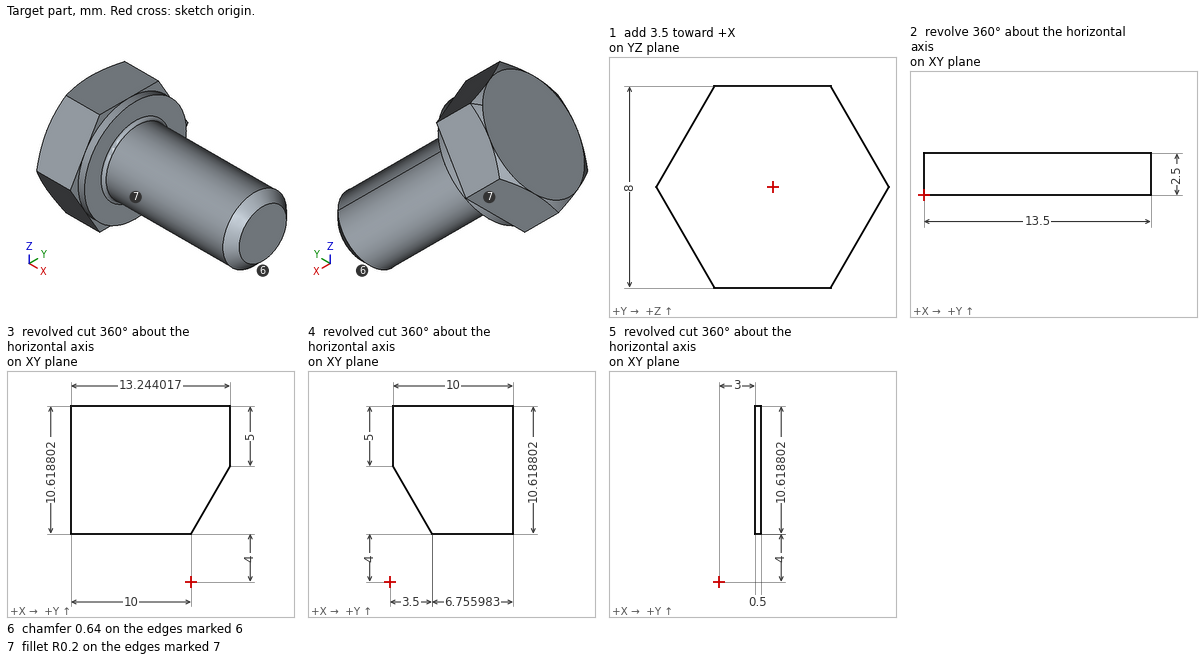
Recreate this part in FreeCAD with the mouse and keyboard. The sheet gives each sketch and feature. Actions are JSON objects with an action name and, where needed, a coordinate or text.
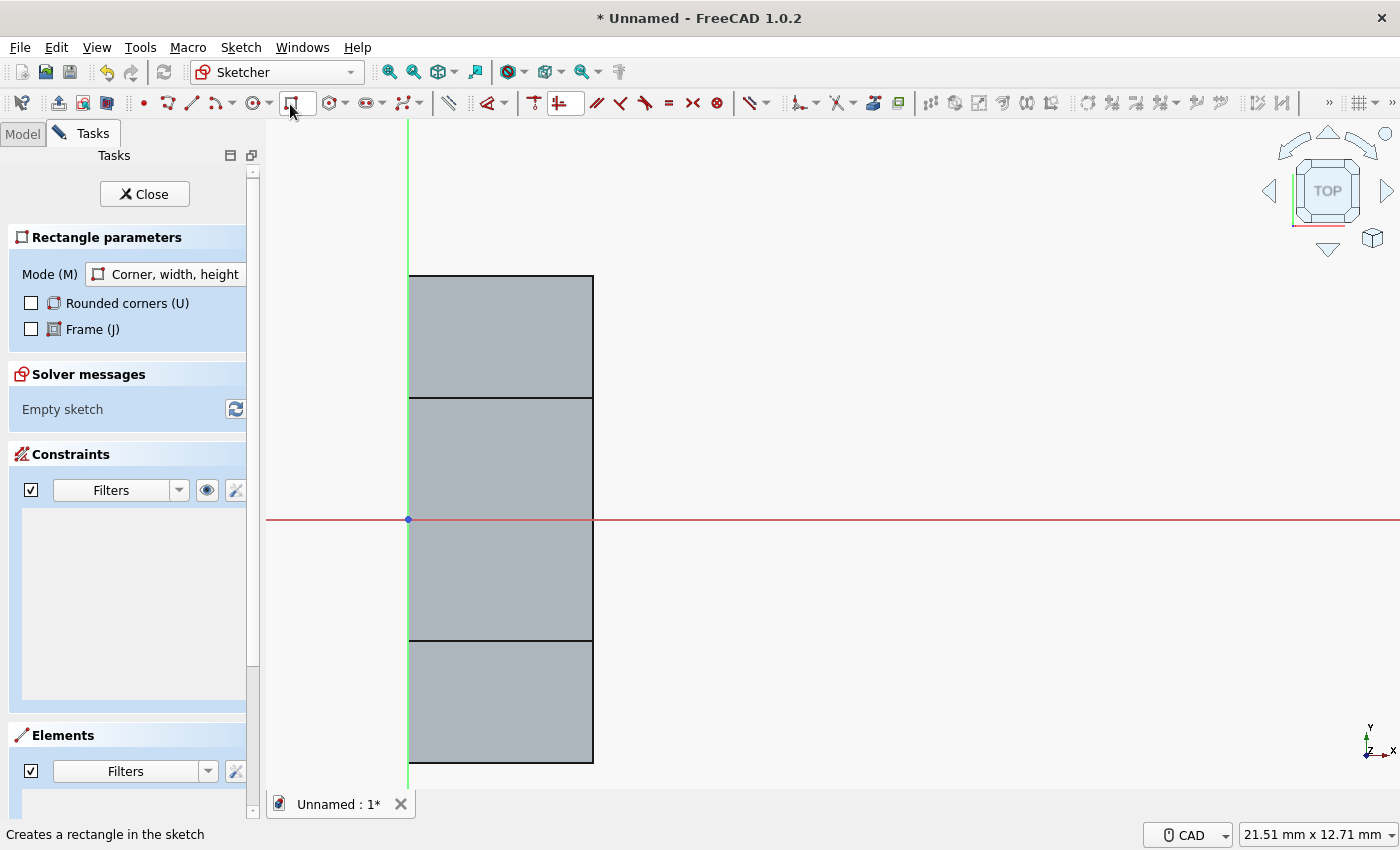
{"action": "left_click", "coordinate": [408, 520]}
{"action": "mouse_move", "coordinate": [1120, 388]}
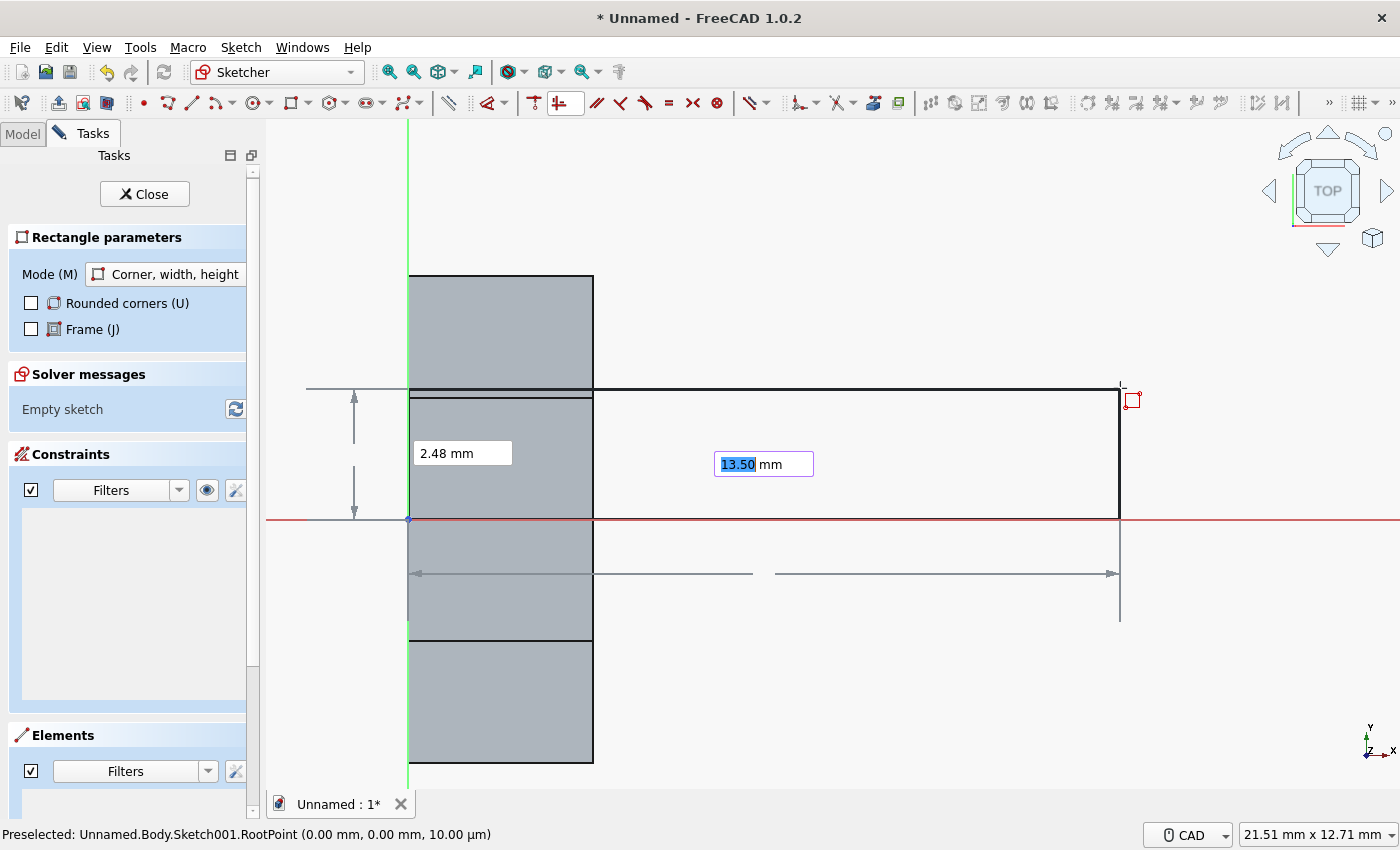
{"action": "type", "text": "13.5"}
{"action": "key", "text": "Tab"}
{"action": "type", "text": "2.5"}
{"action": "key", "text": "Return"}
{"action": "key", "text": "Escape"}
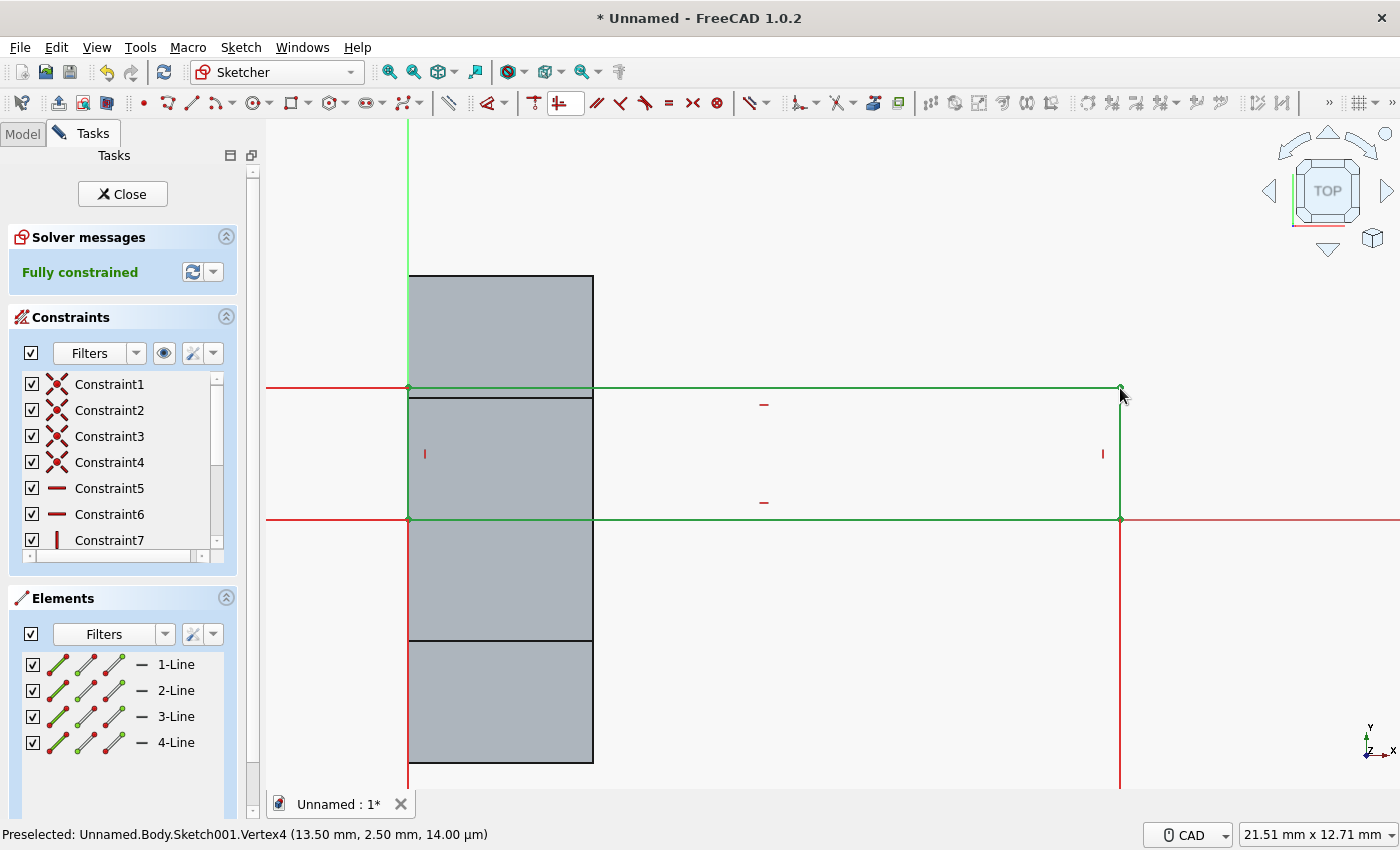
{"action": "left_click", "coordinate": [123, 194]}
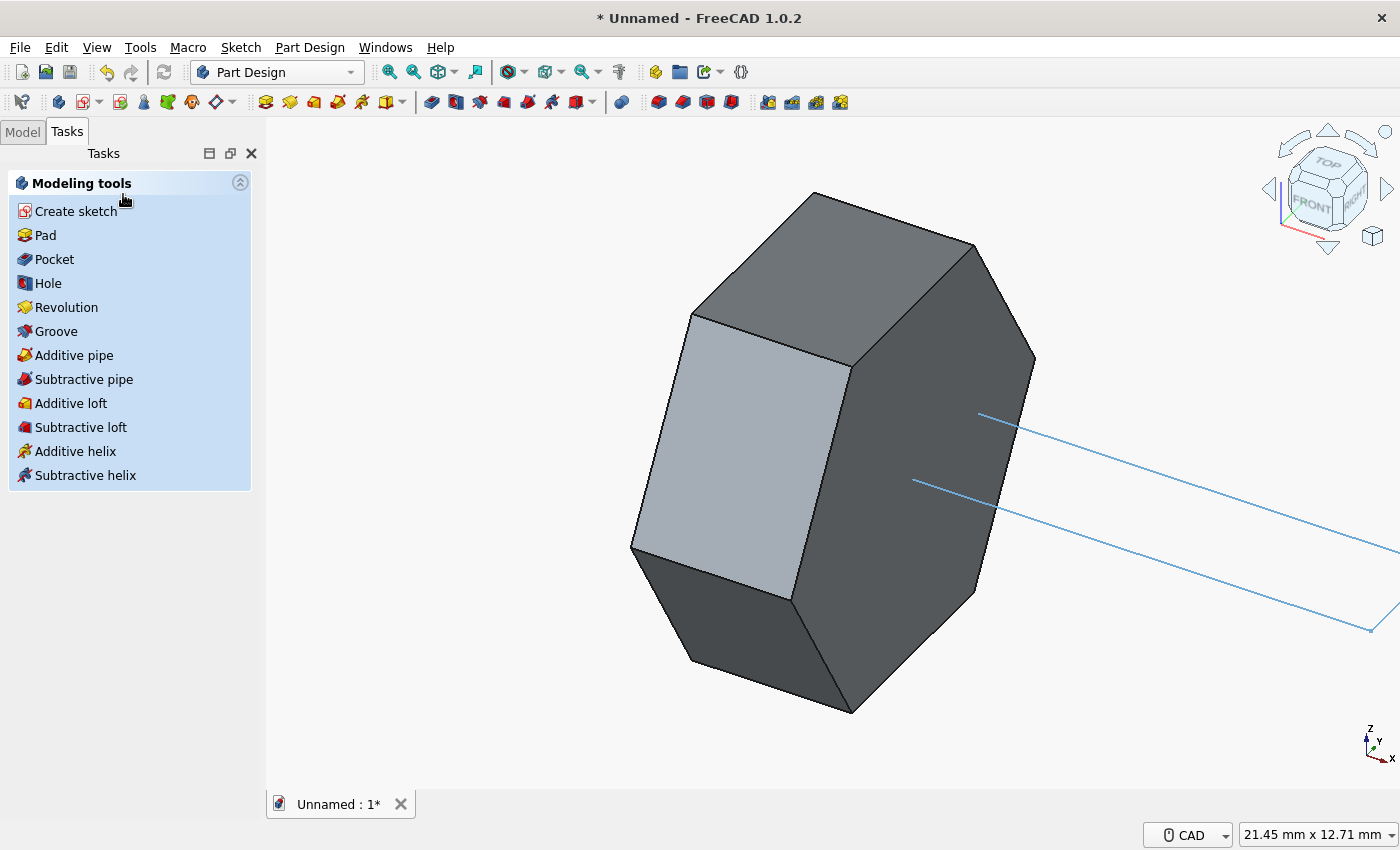
{"action": "left_click", "coordinate": [290, 102]}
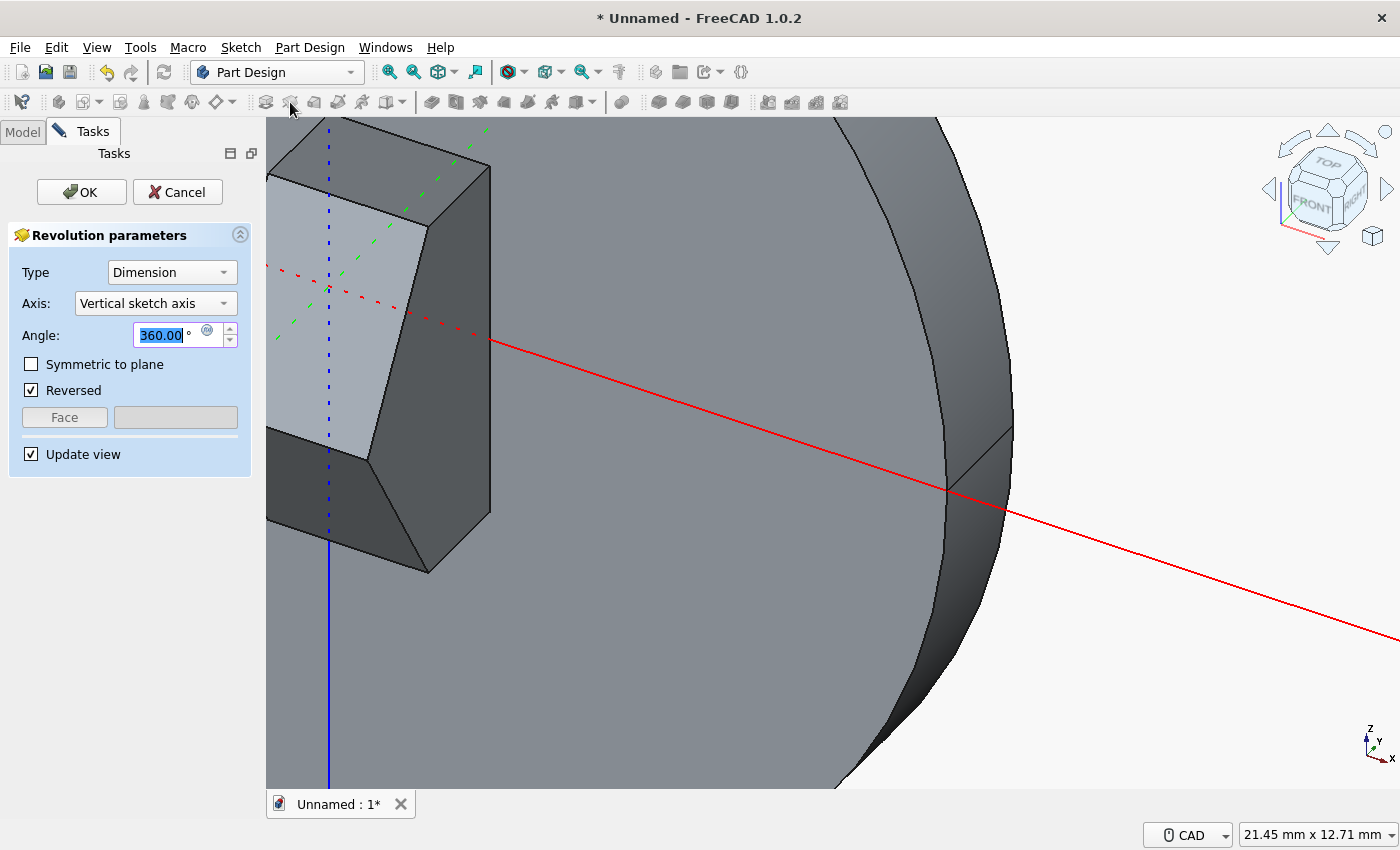
{"action": "left_click", "coordinate": [156, 304]}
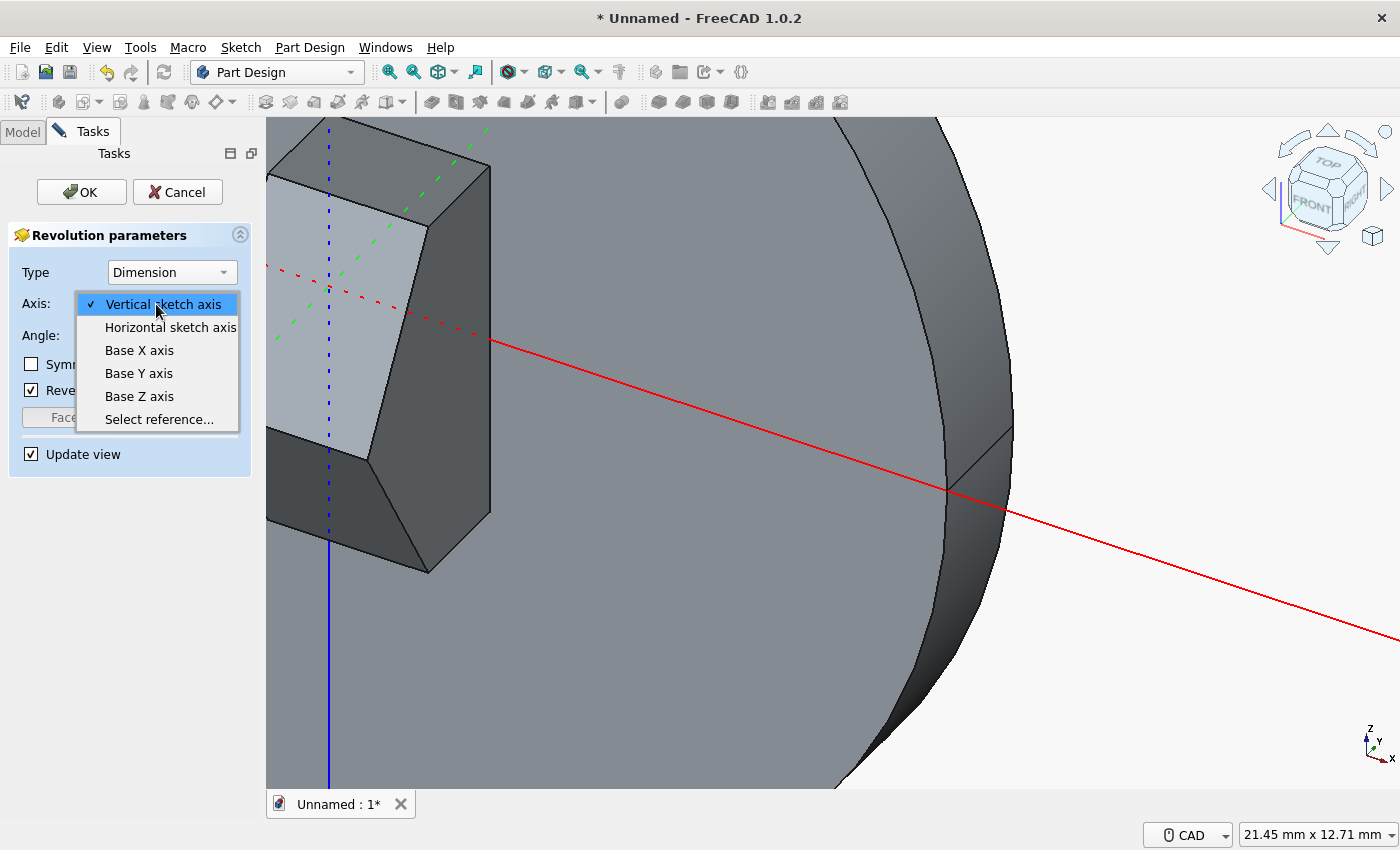
{"action": "left_click", "coordinate": [156, 328]}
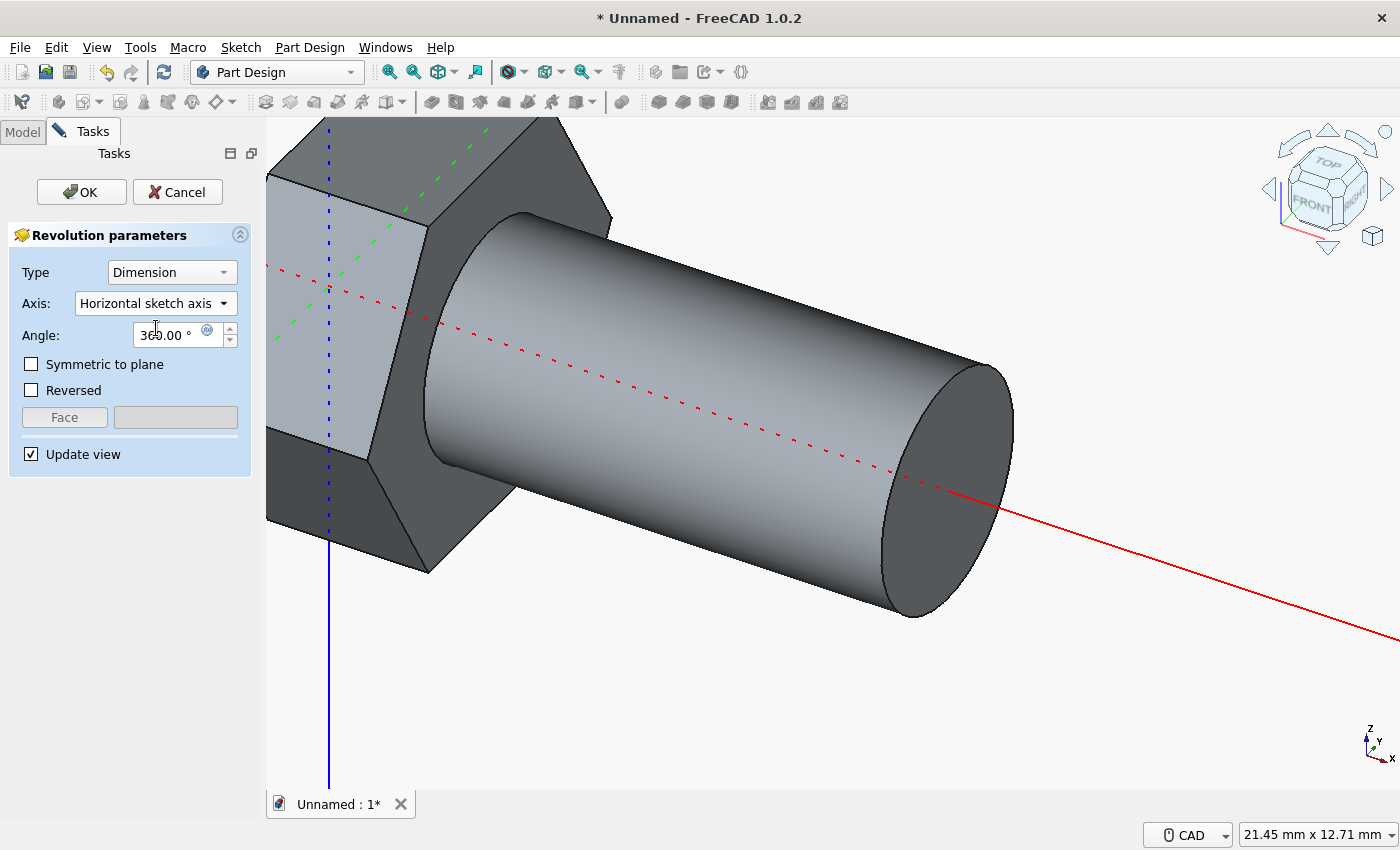
{"action": "left_click", "coordinate": [82, 192]}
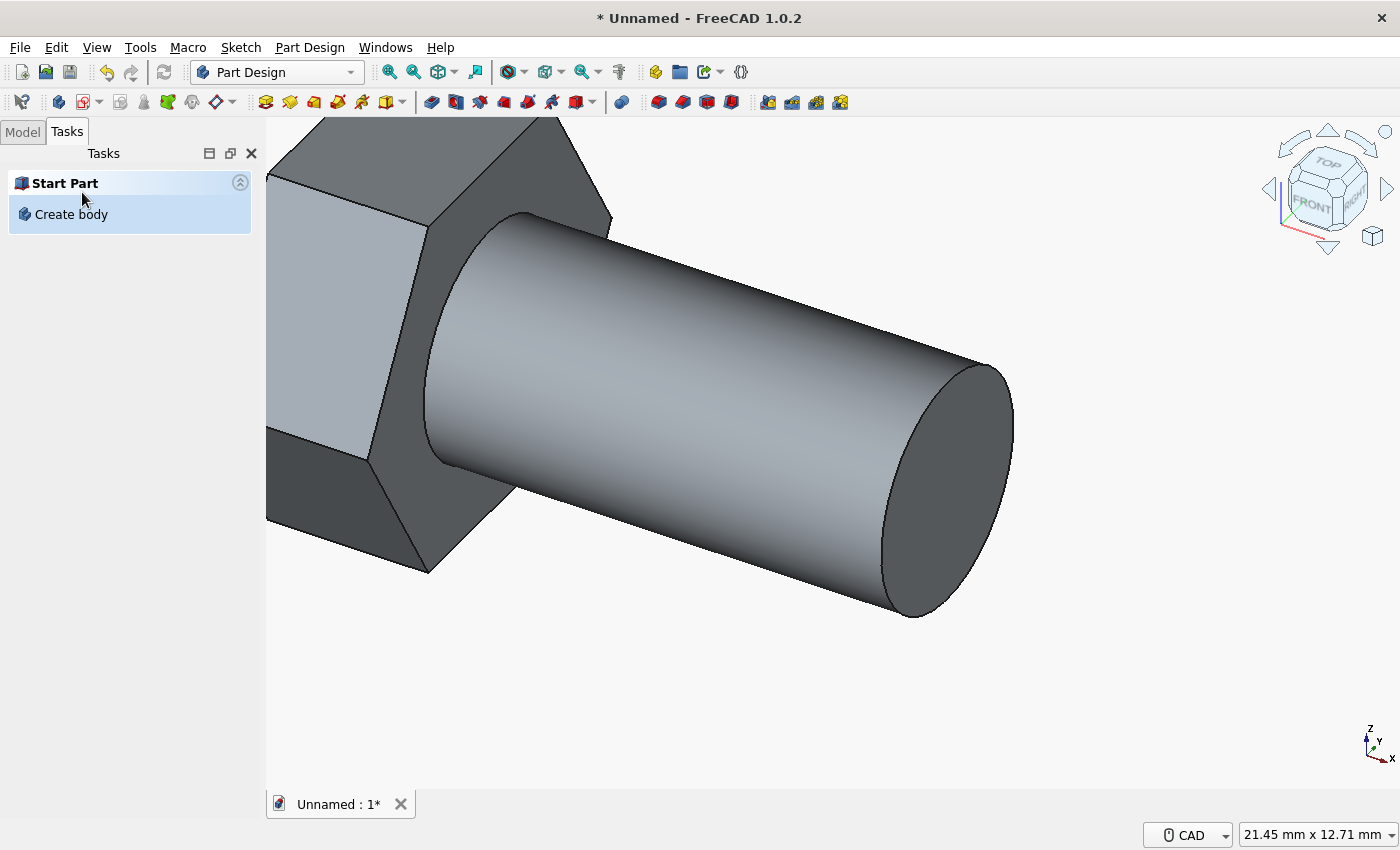
{"action": "left_click", "coordinate": [390, 72]}